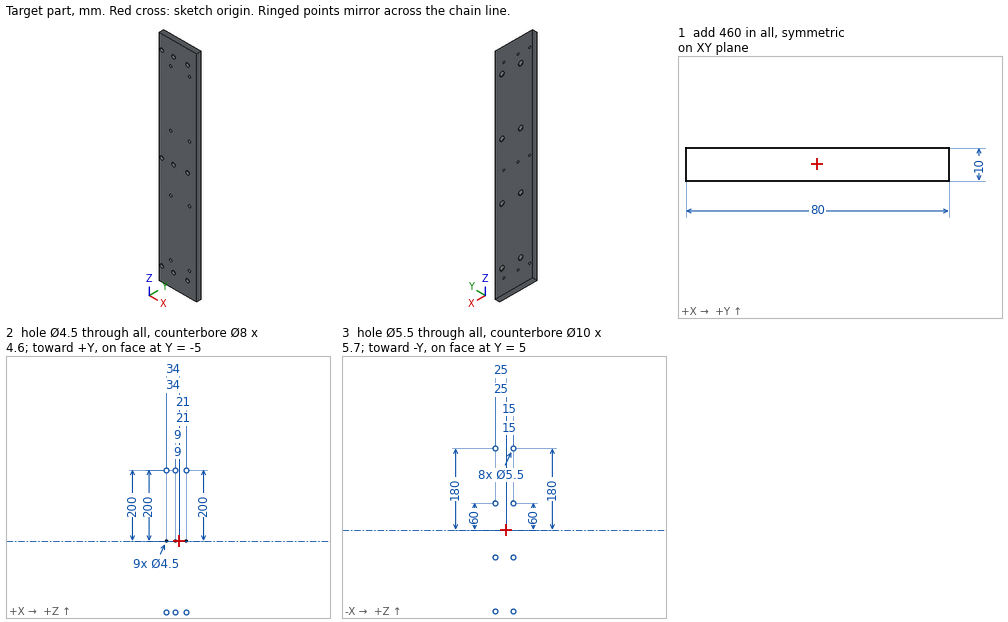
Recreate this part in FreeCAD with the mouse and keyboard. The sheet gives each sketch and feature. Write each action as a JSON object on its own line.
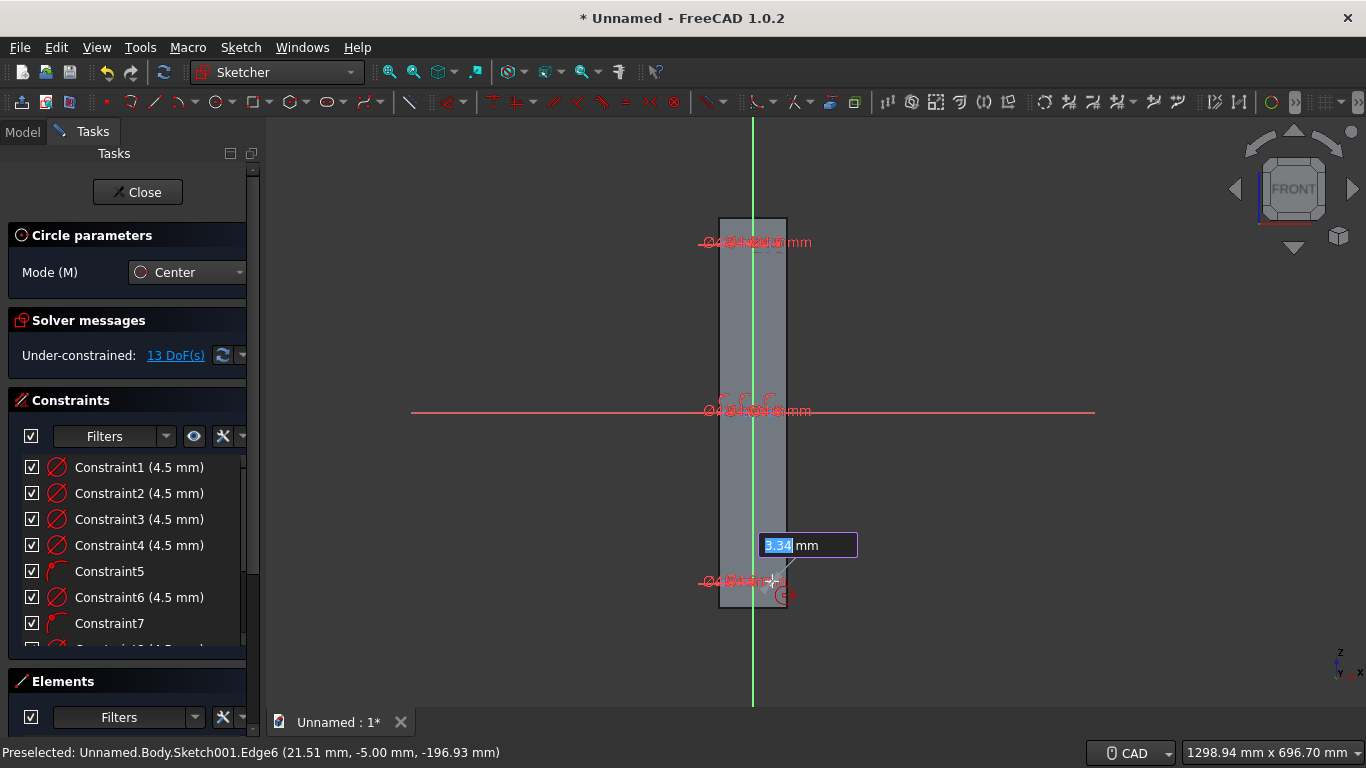
{"action": "type", "text": "4.5"}
{"action": "key", "text": "Return"}
{"action": "key", "text": "Escape"}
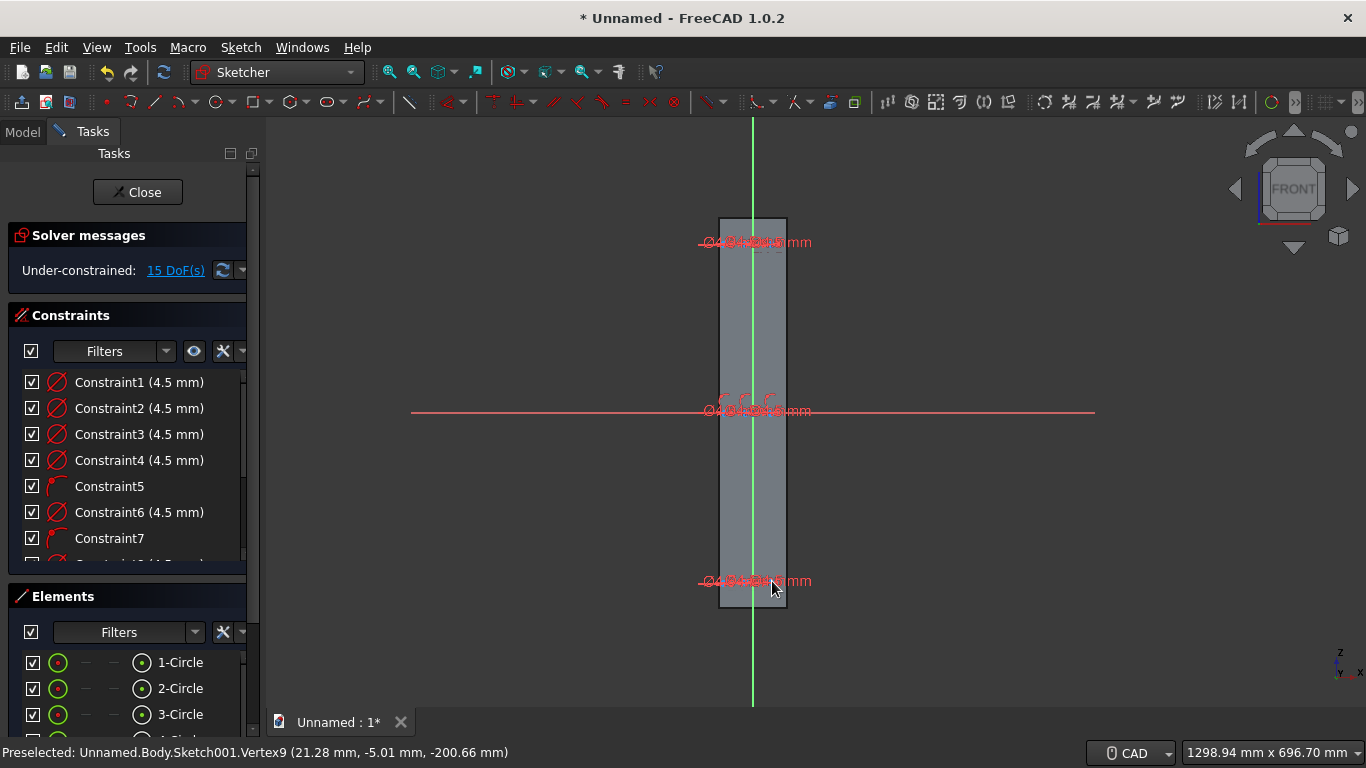
{"action": "left_click", "coordinate": [724, 245]}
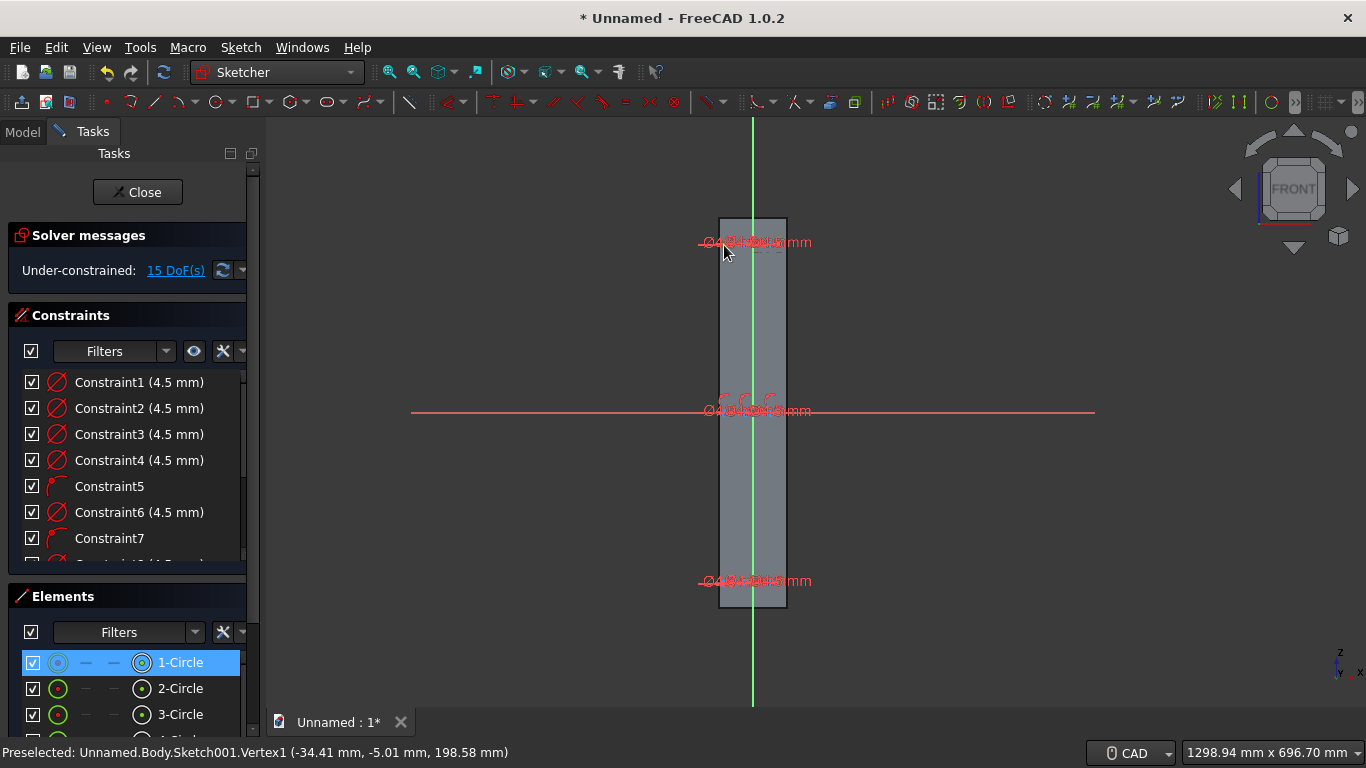
{"action": "left_click", "coordinate": [724, 584]}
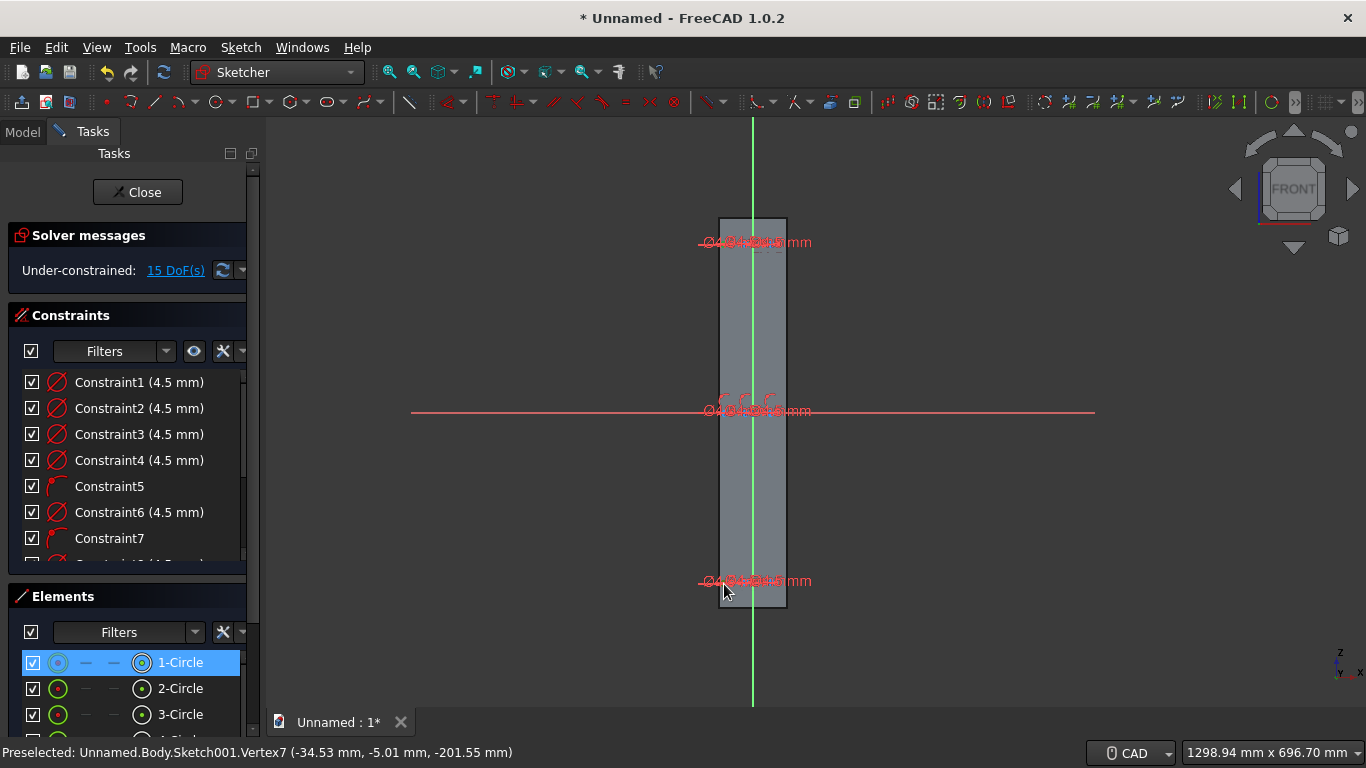
{"action": "left_click", "coordinate": [424, 413]}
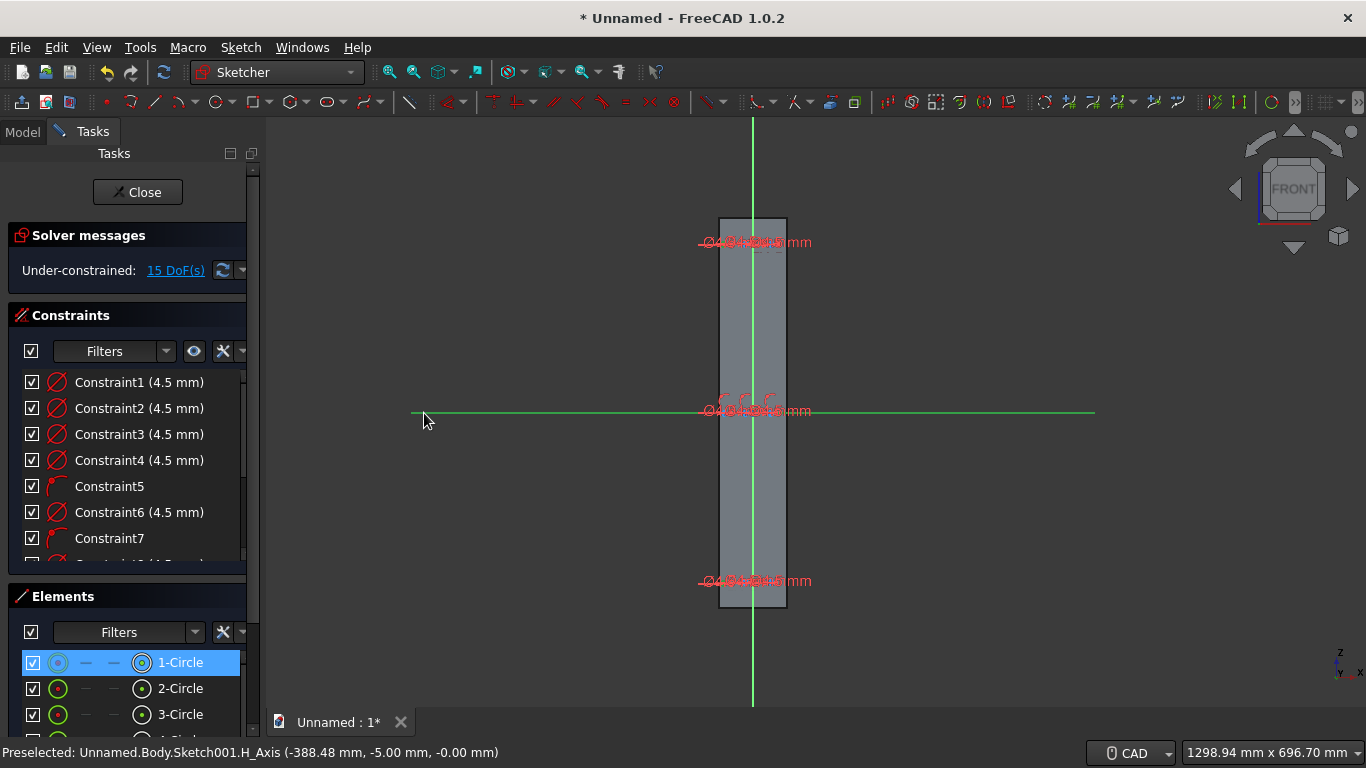
{"action": "key", "text": "s"}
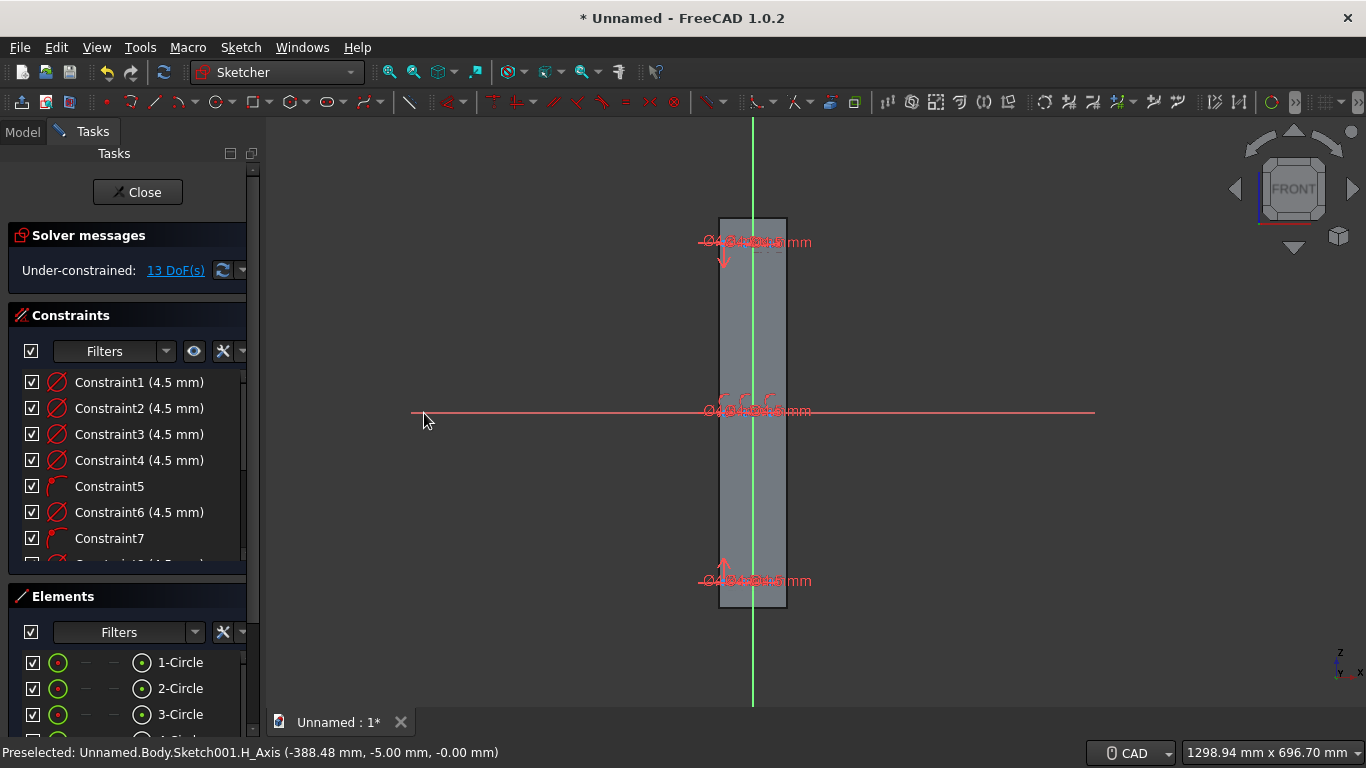
{"action": "left_click", "coordinate": [745, 244]}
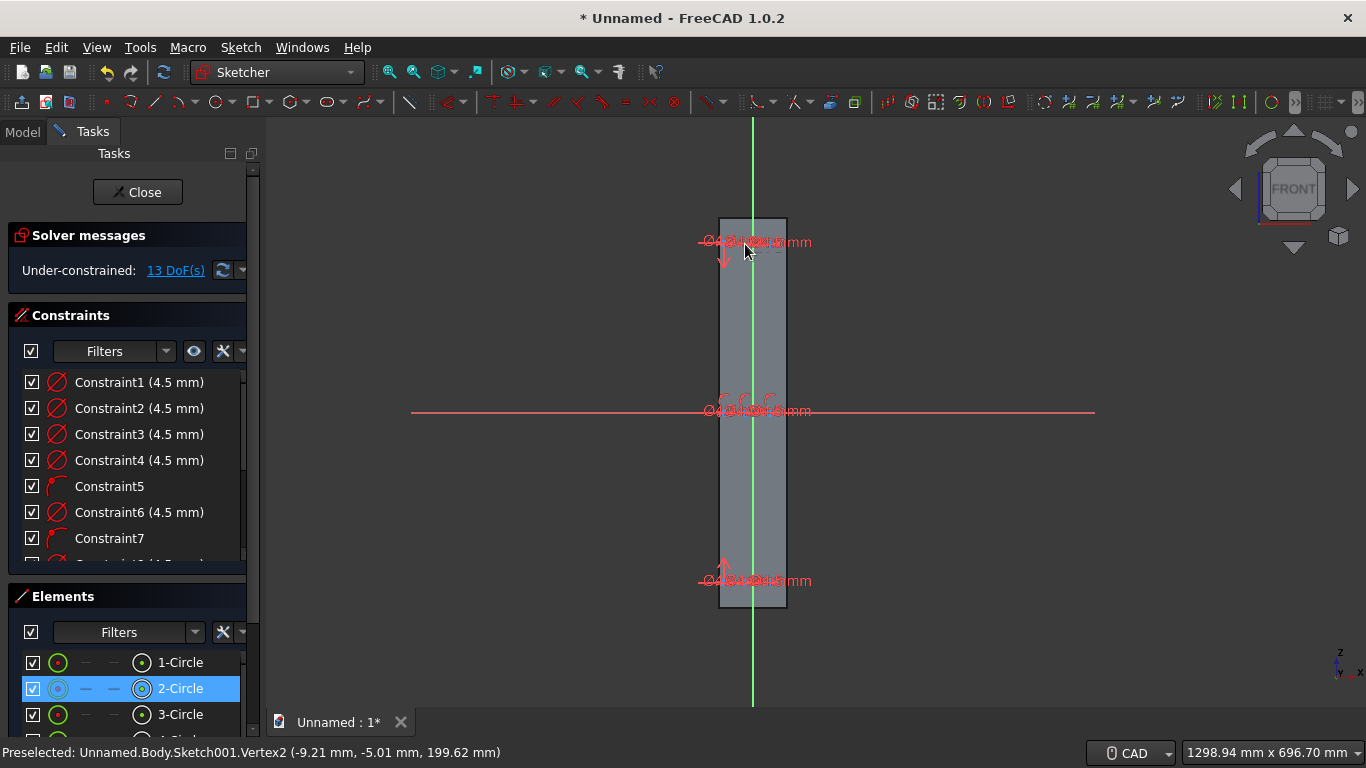
{"action": "left_click", "coordinate": [746, 583]}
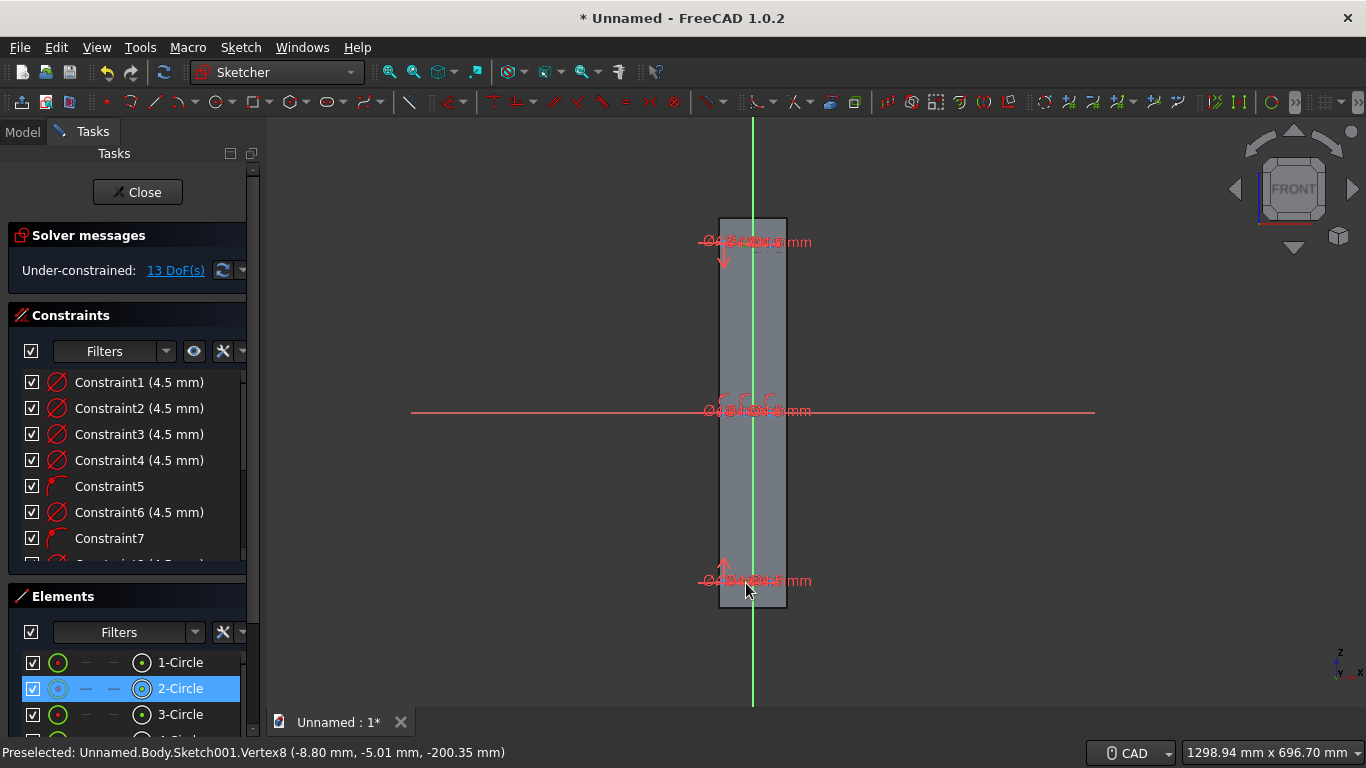
{"action": "left_click", "coordinate": [424, 413]}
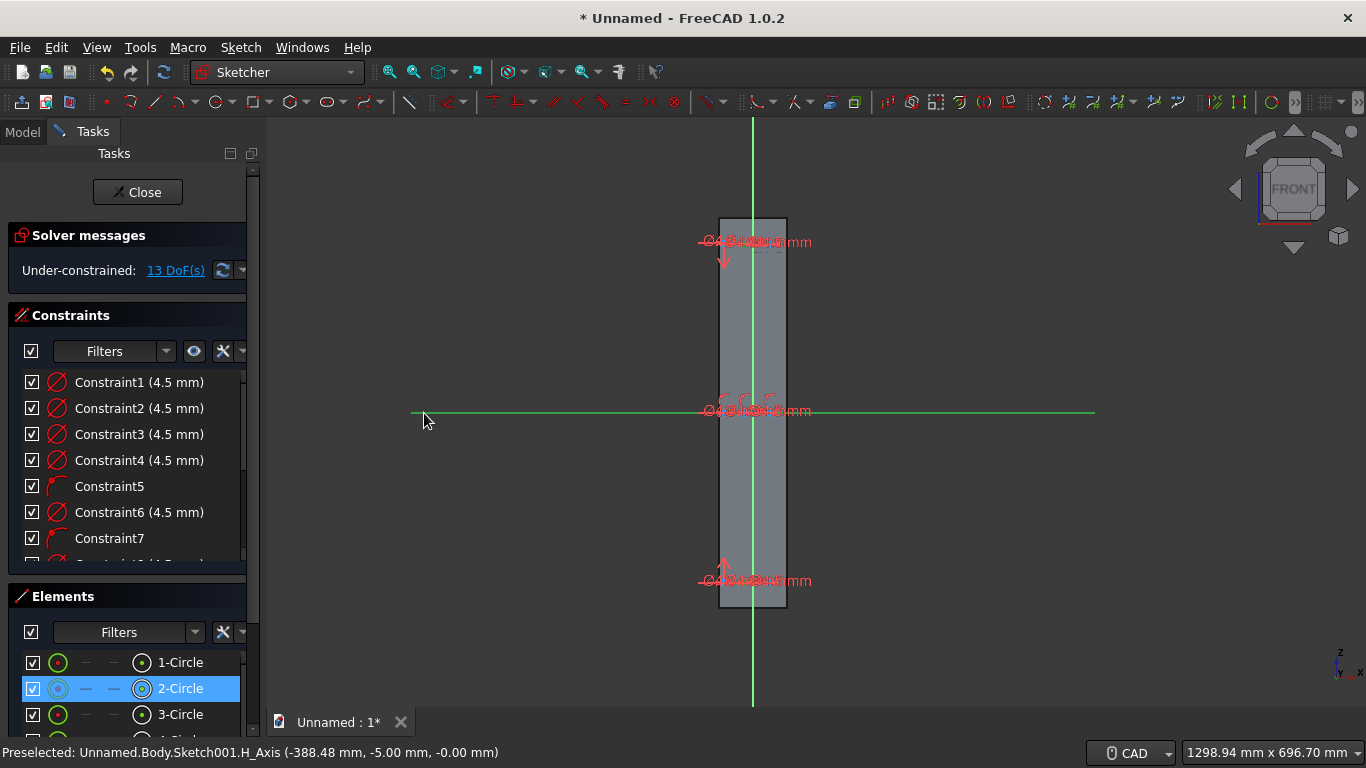
{"action": "key", "text": "s"}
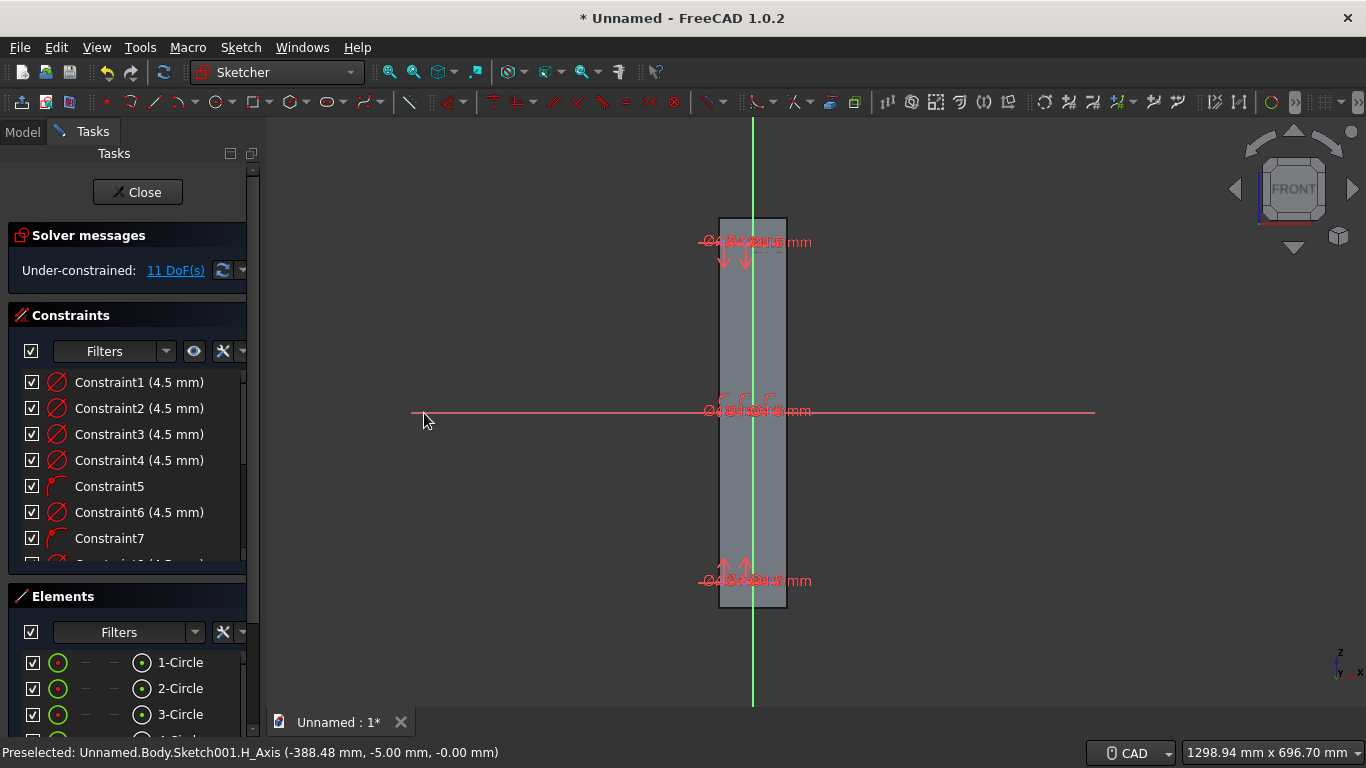
{"action": "left_click", "coordinate": [771, 245]}